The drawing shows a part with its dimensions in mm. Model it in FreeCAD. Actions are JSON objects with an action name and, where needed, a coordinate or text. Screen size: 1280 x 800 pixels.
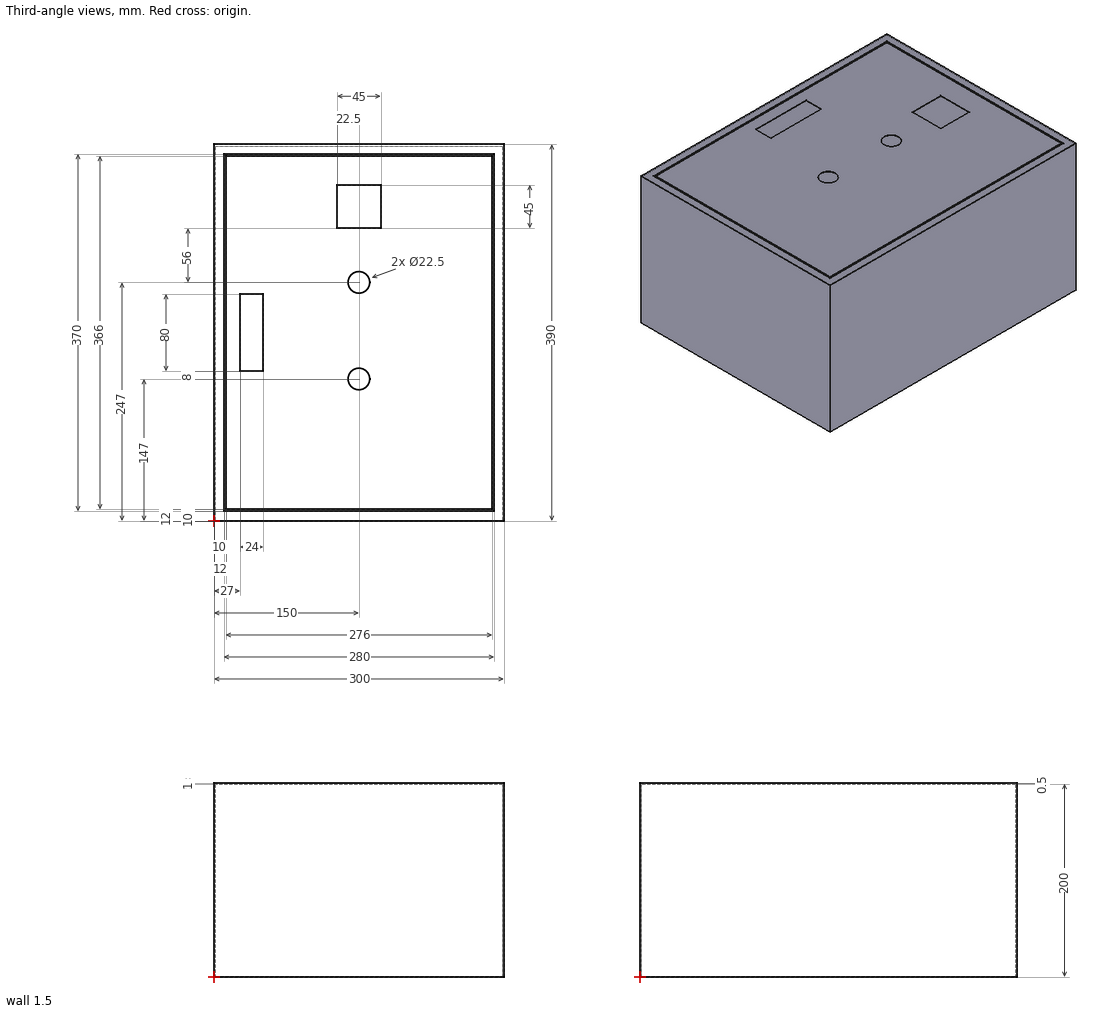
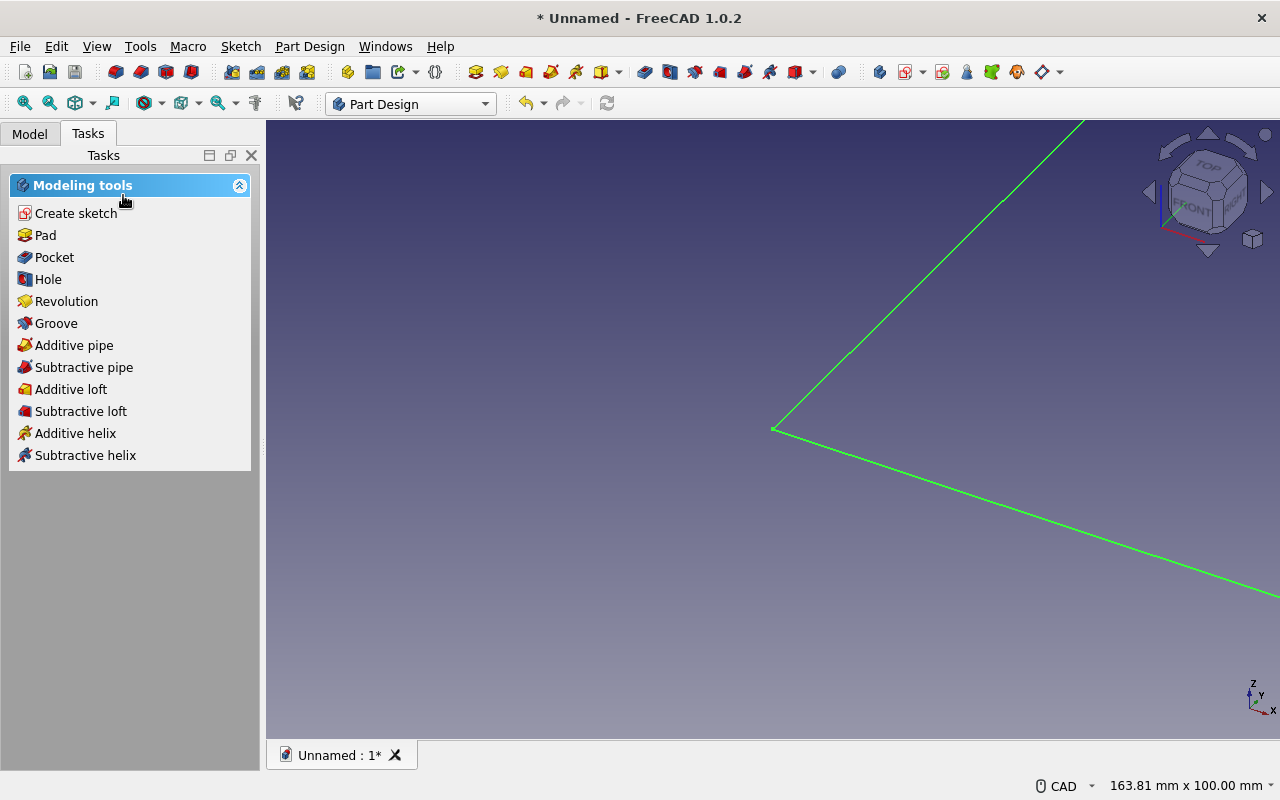
{"action": "left_click", "coordinate": [476, 72]}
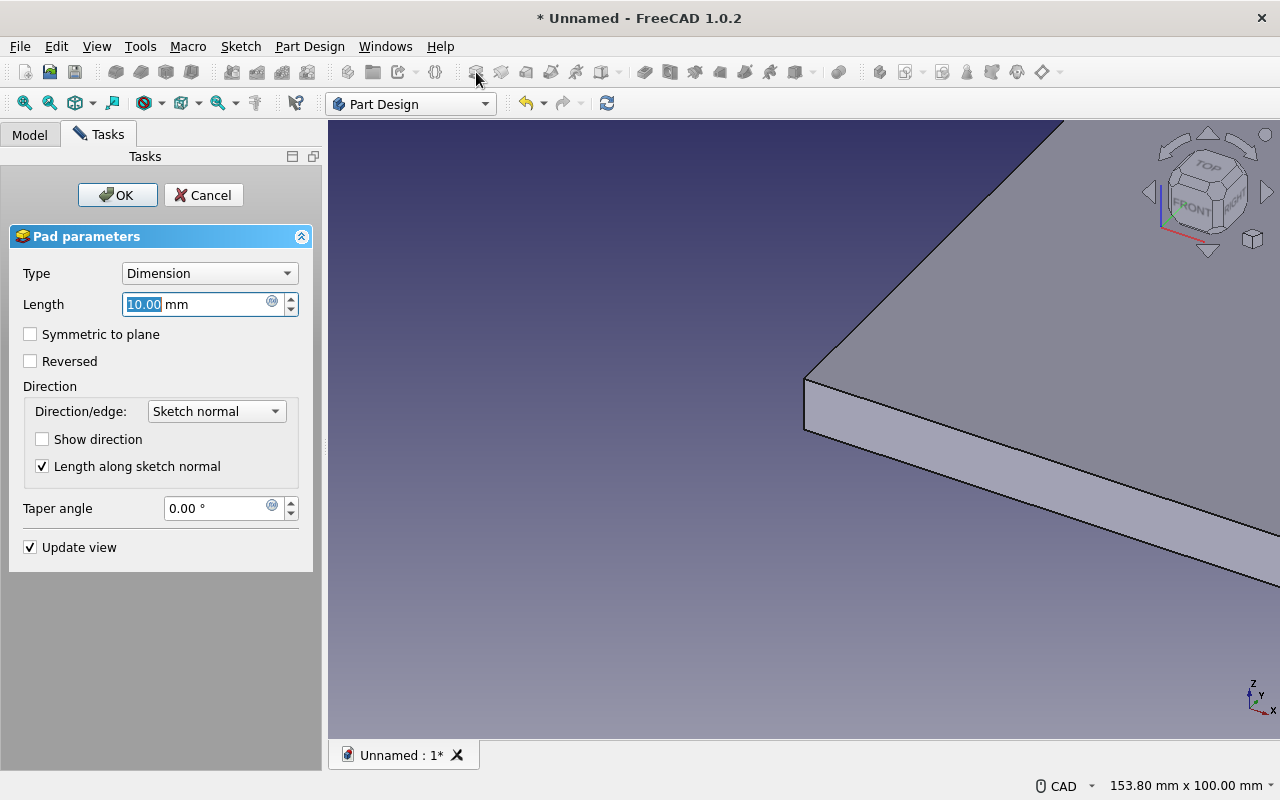
{"action": "type", "text": "200"}
{"action": "key", "text": "Tab"}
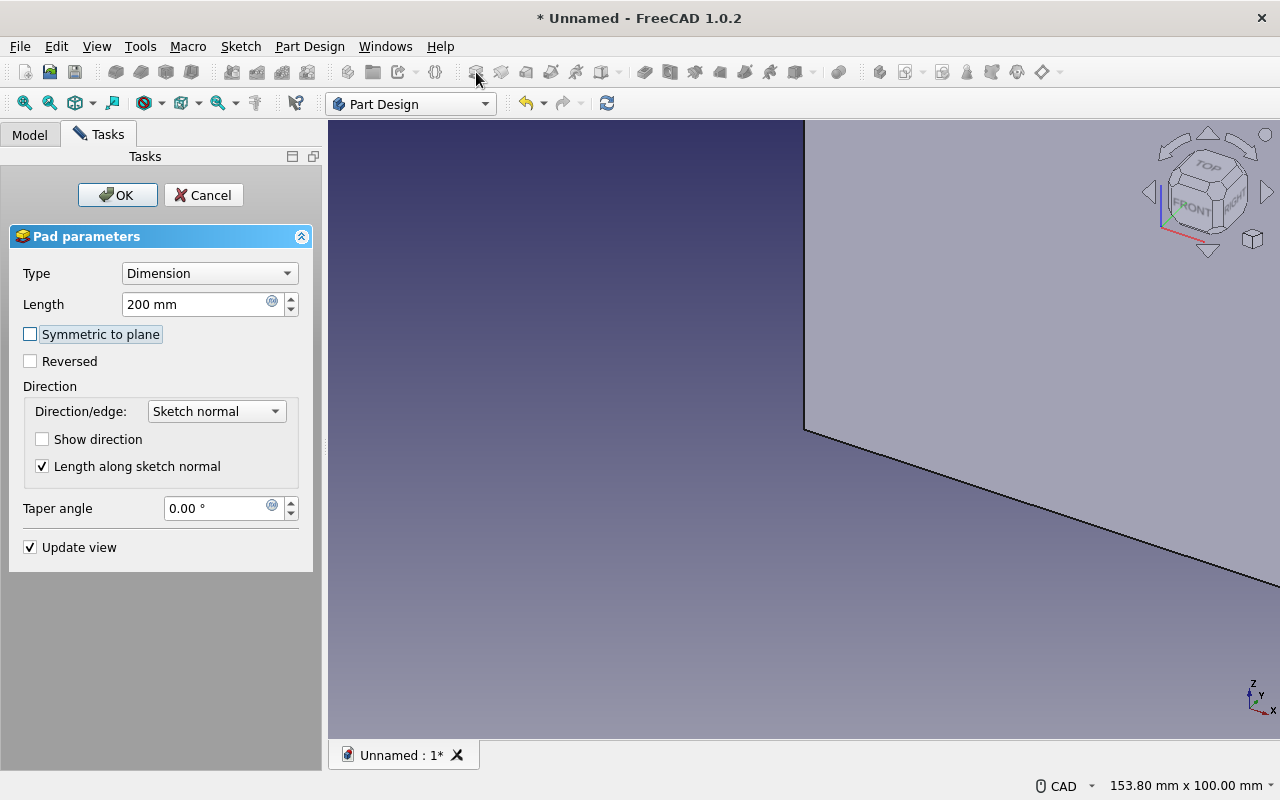
{"action": "left_click", "coordinate": [118, 195]}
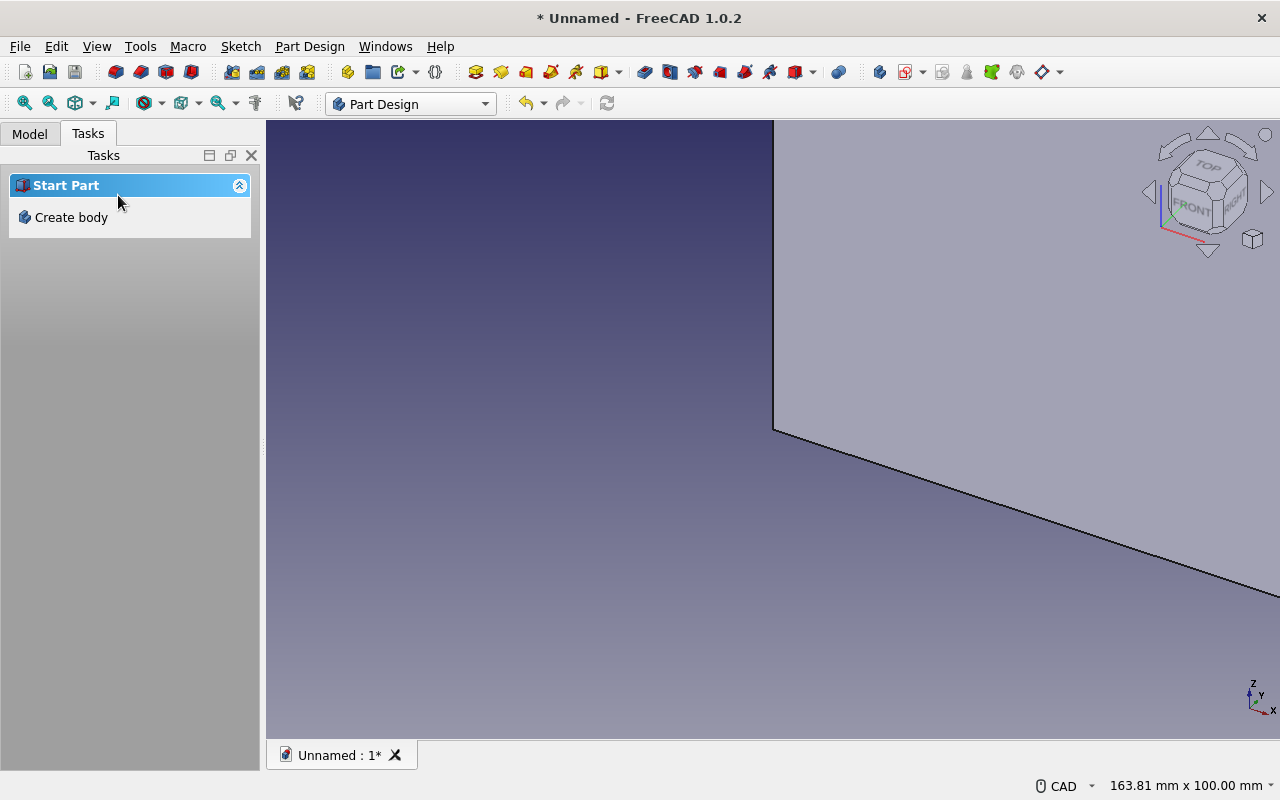
{"action": "left_click", "coordinate": [25, 104]}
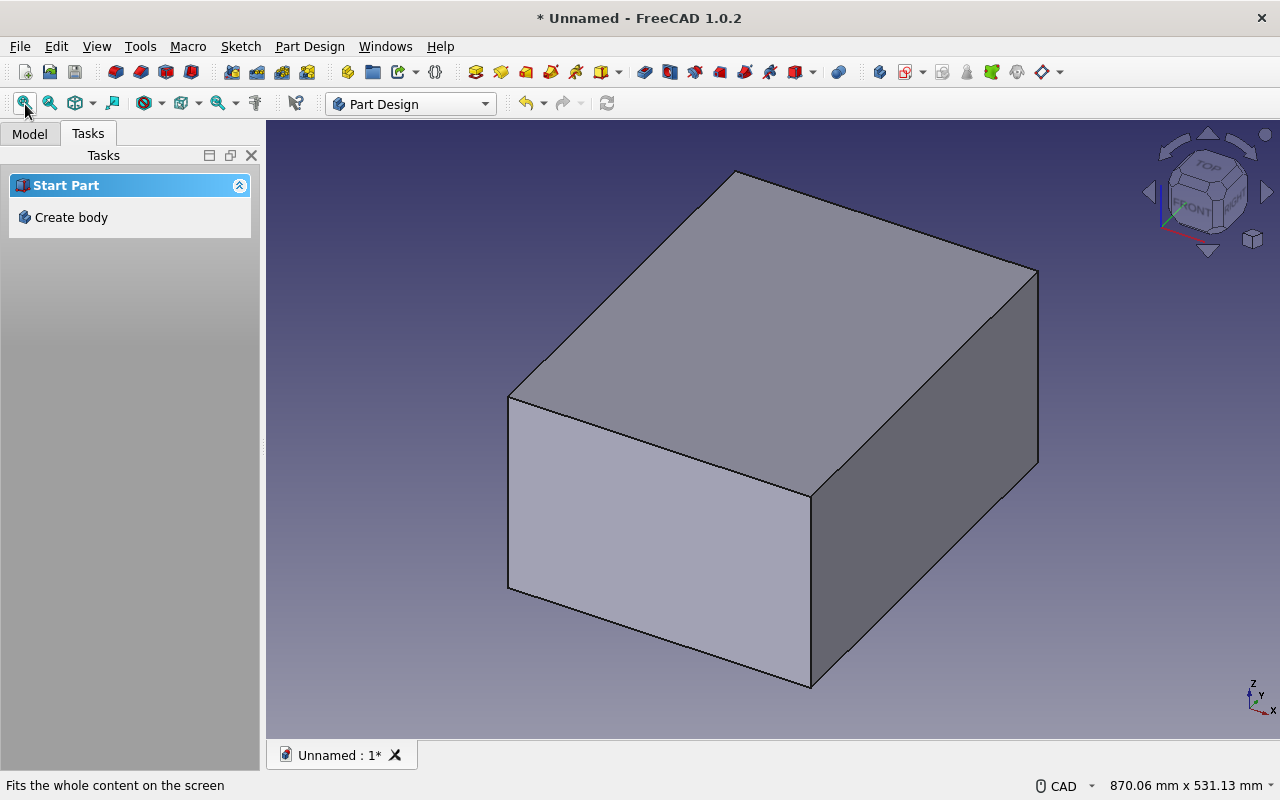
{"action": "left_click", "coordinate": [773, 333]}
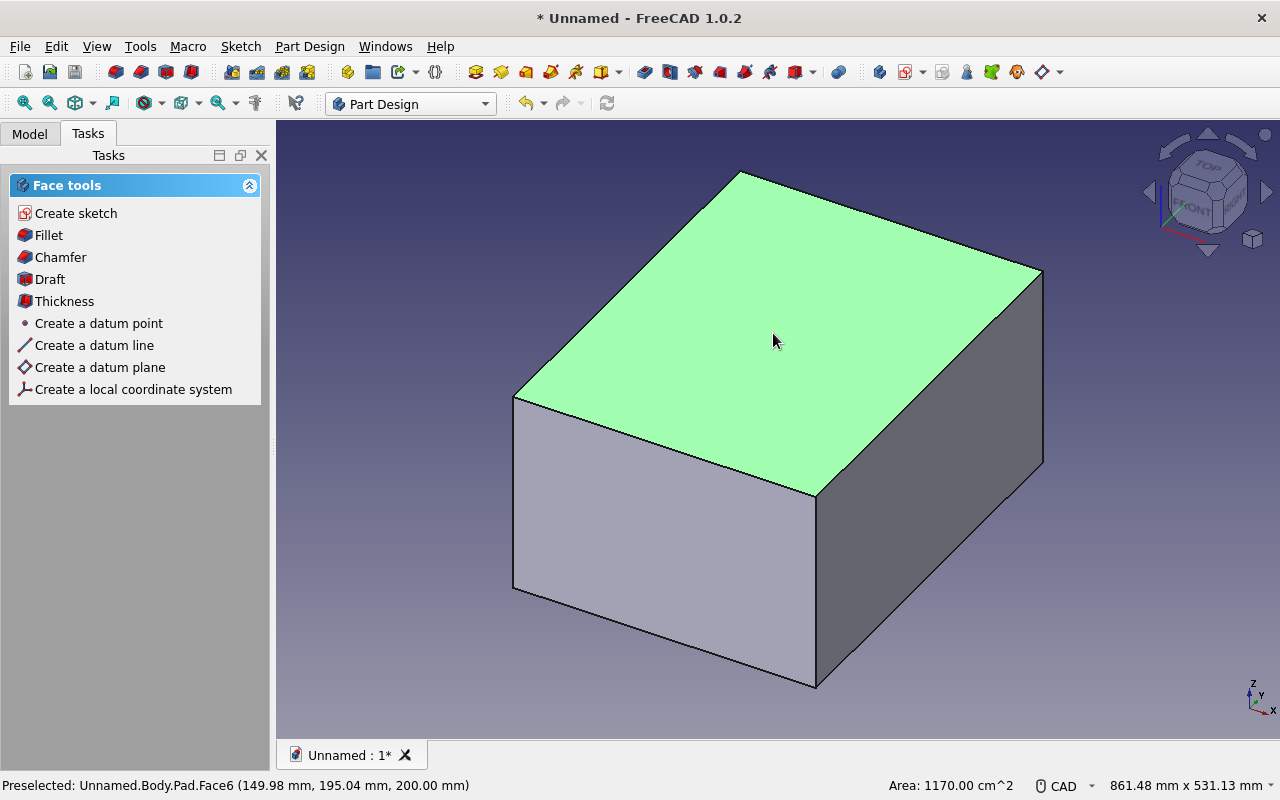
{"action": "left_click", "coordinate": [191, 72]}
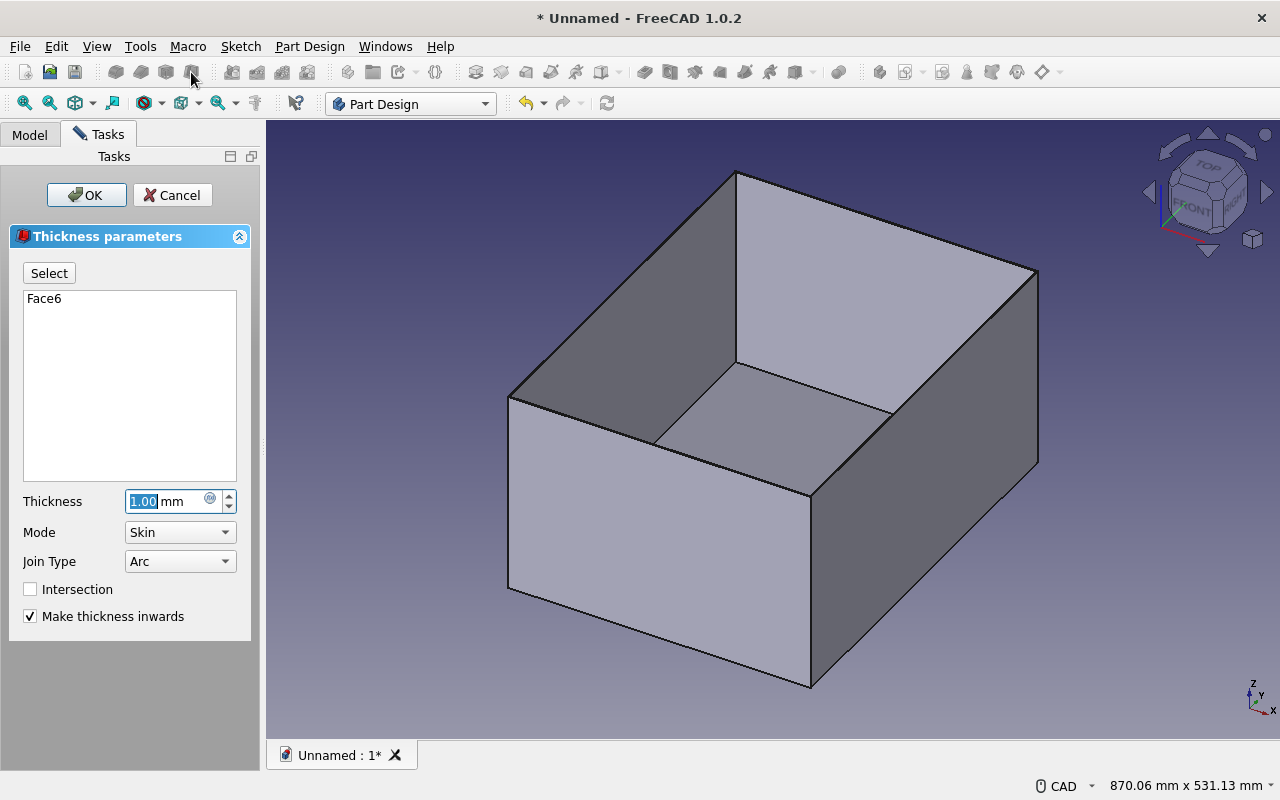
{"action": "type", "text": "1.5"}
{"action": "key", "text": "Tab"}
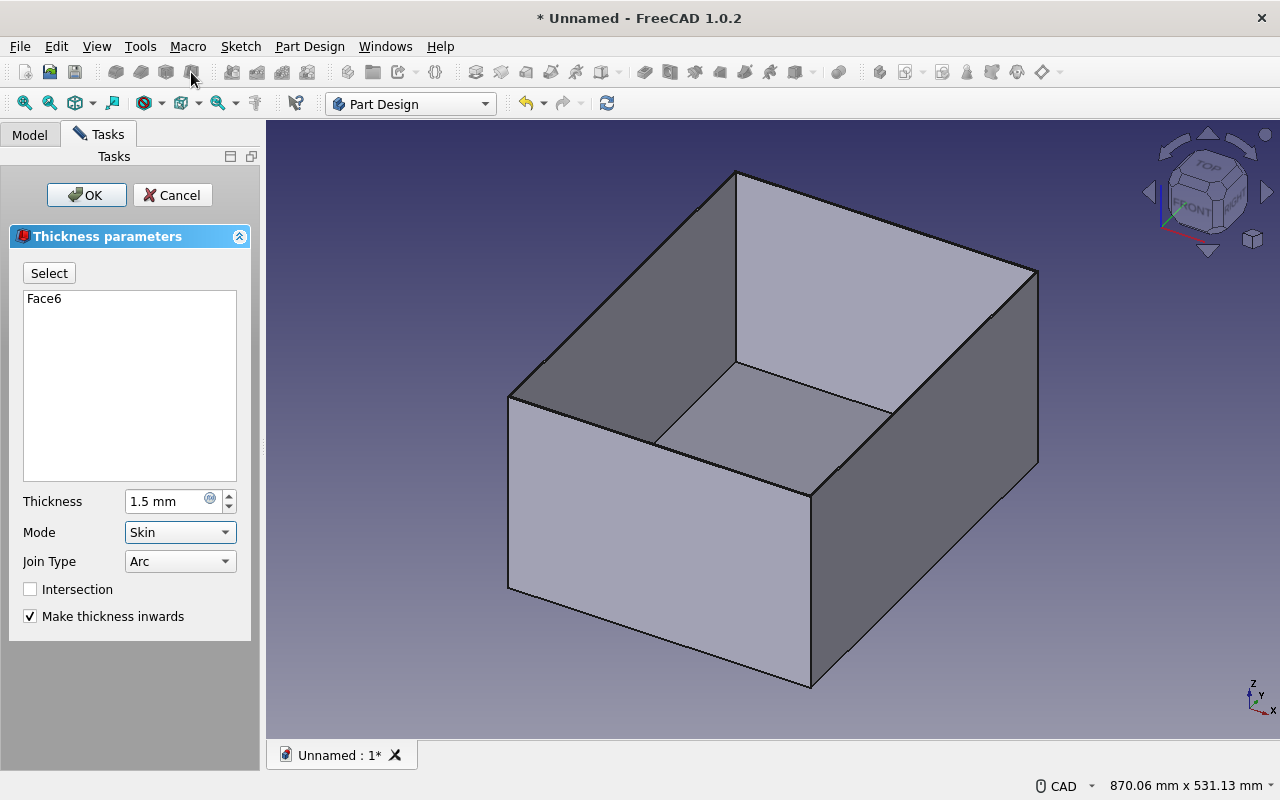
{"action": "left_click", "coordinate": [181, 562]}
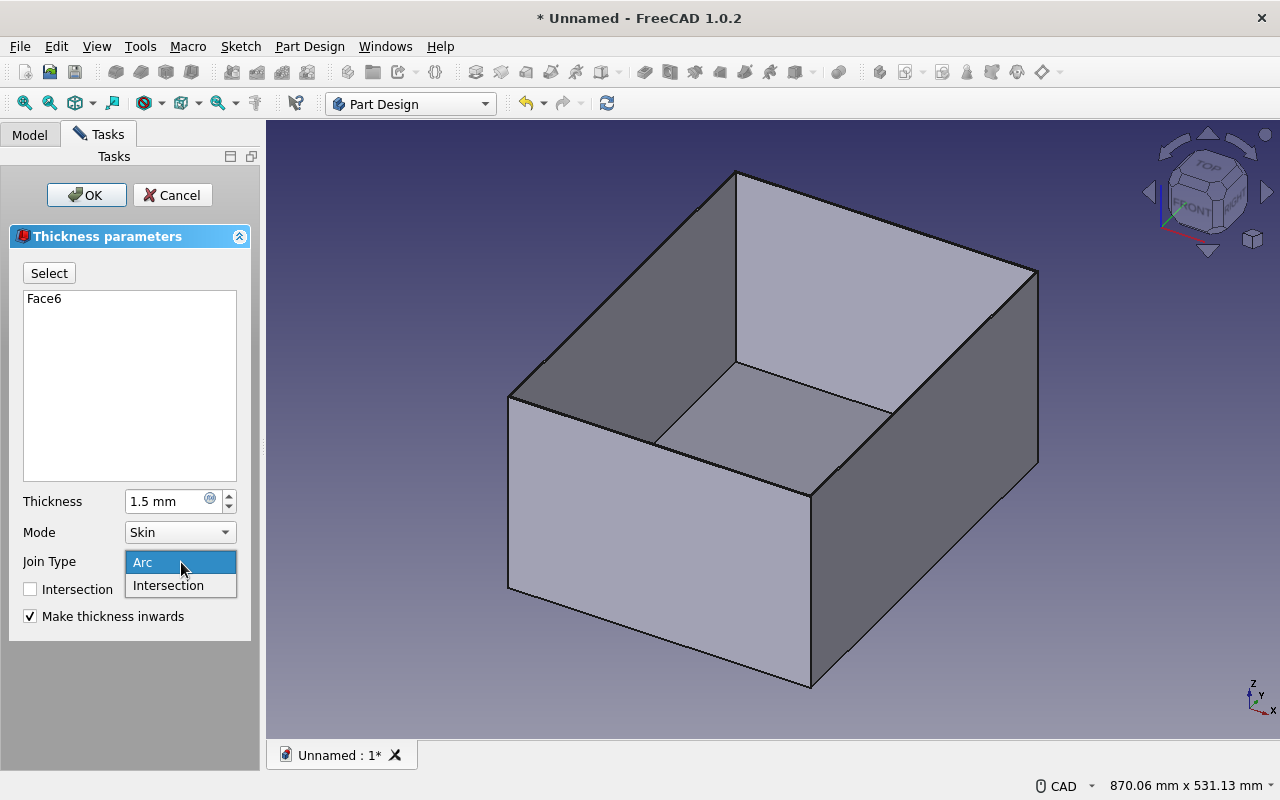
{"action": "left_click", "coordinate": [179, 586]}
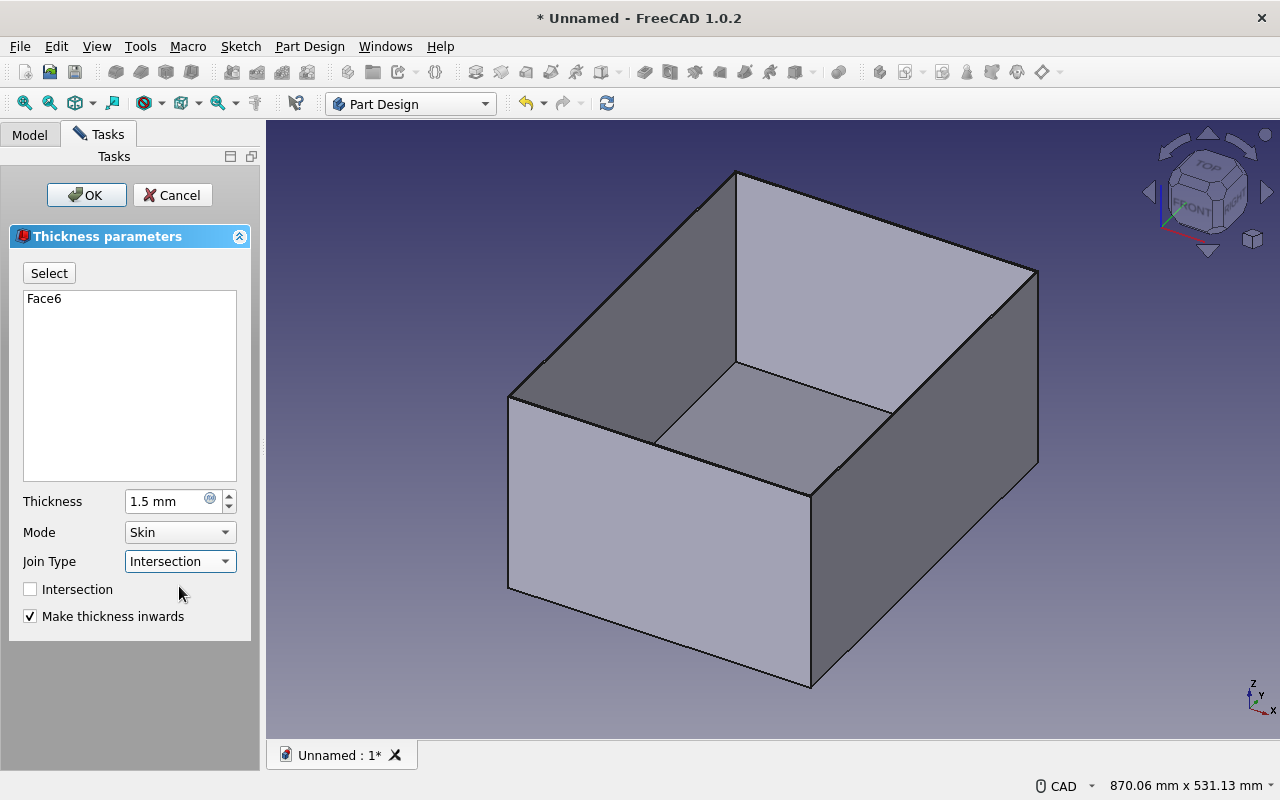
{"action": "left_click", "coordinate": [87, 195]}